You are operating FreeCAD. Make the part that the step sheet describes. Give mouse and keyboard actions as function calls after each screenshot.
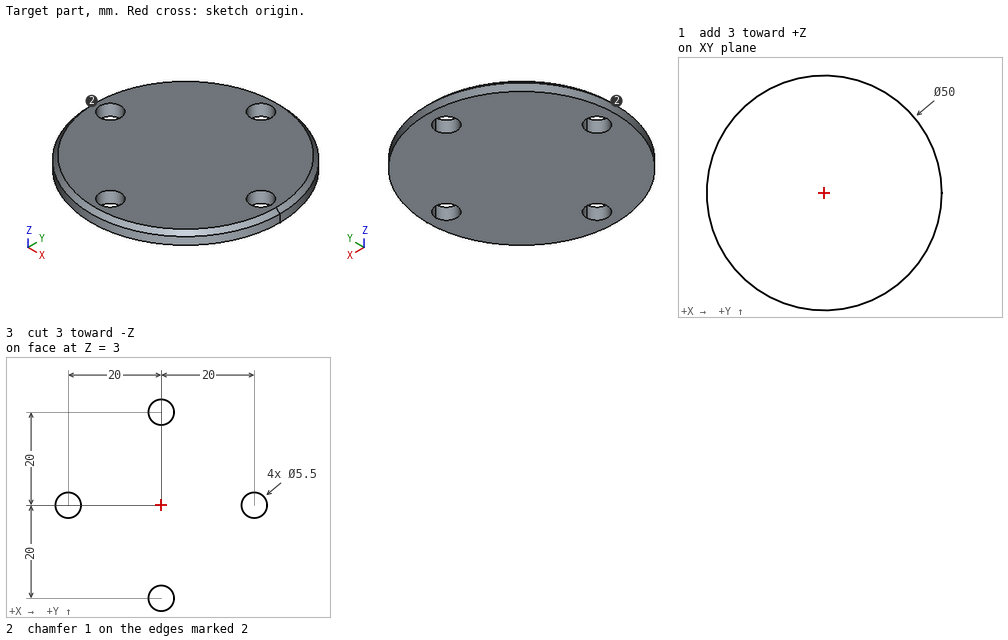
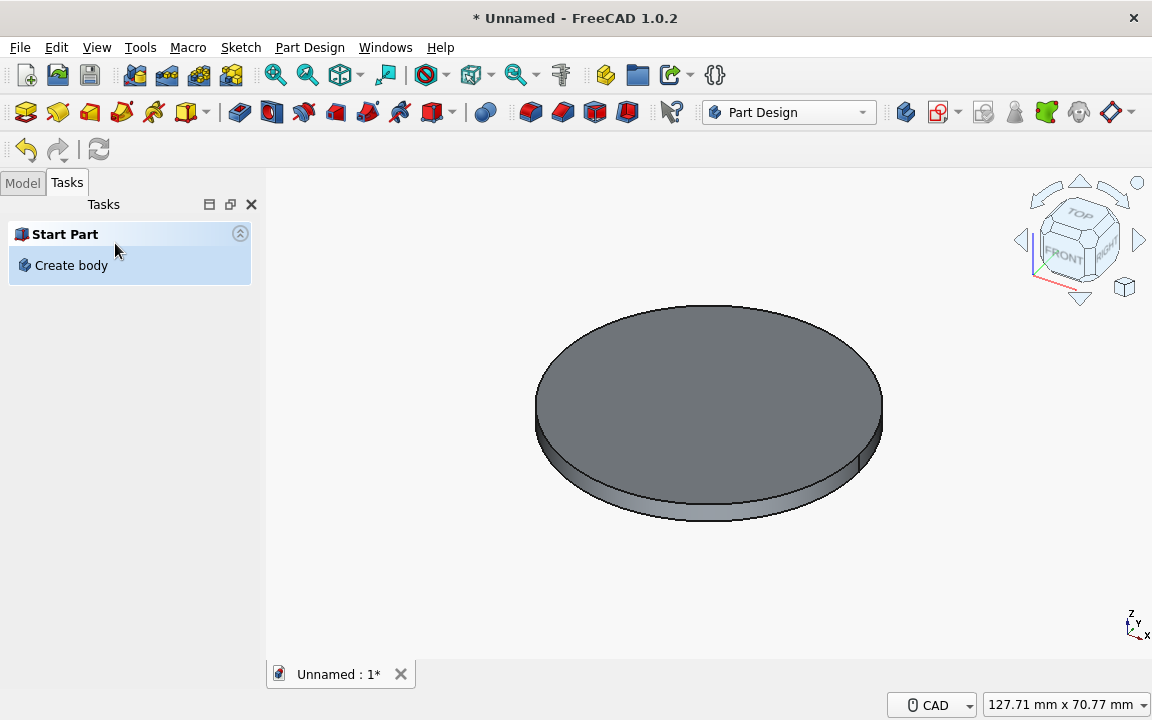
click(537, 414)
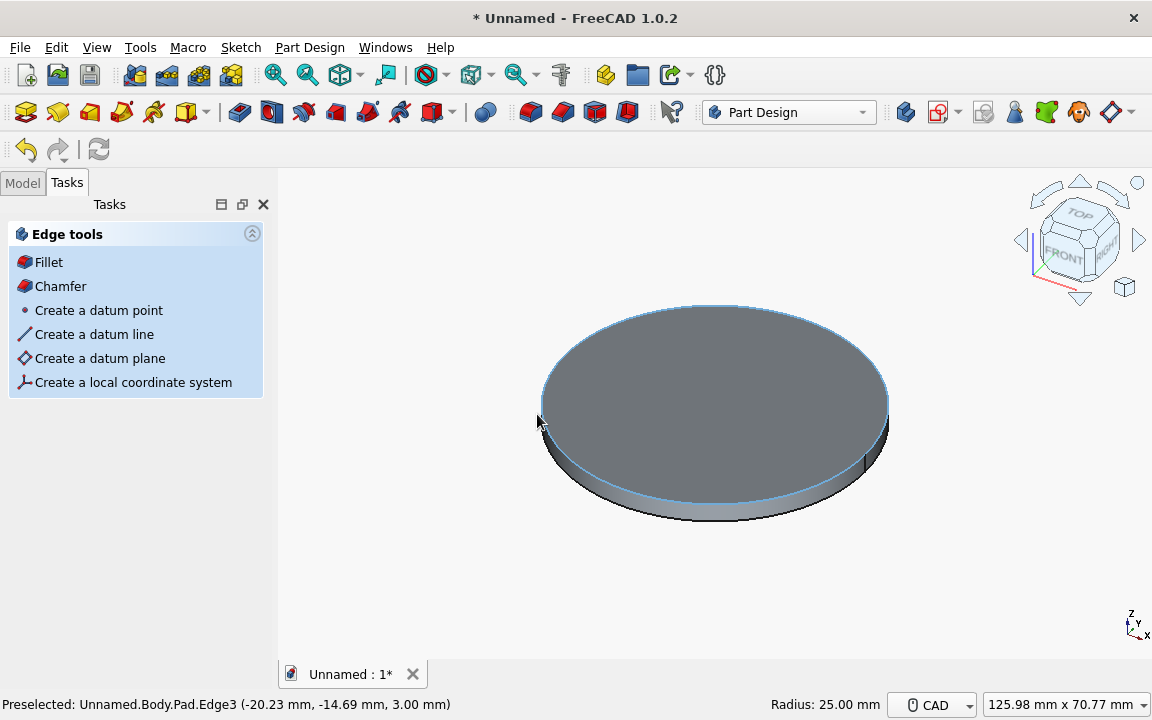
click(564, 112)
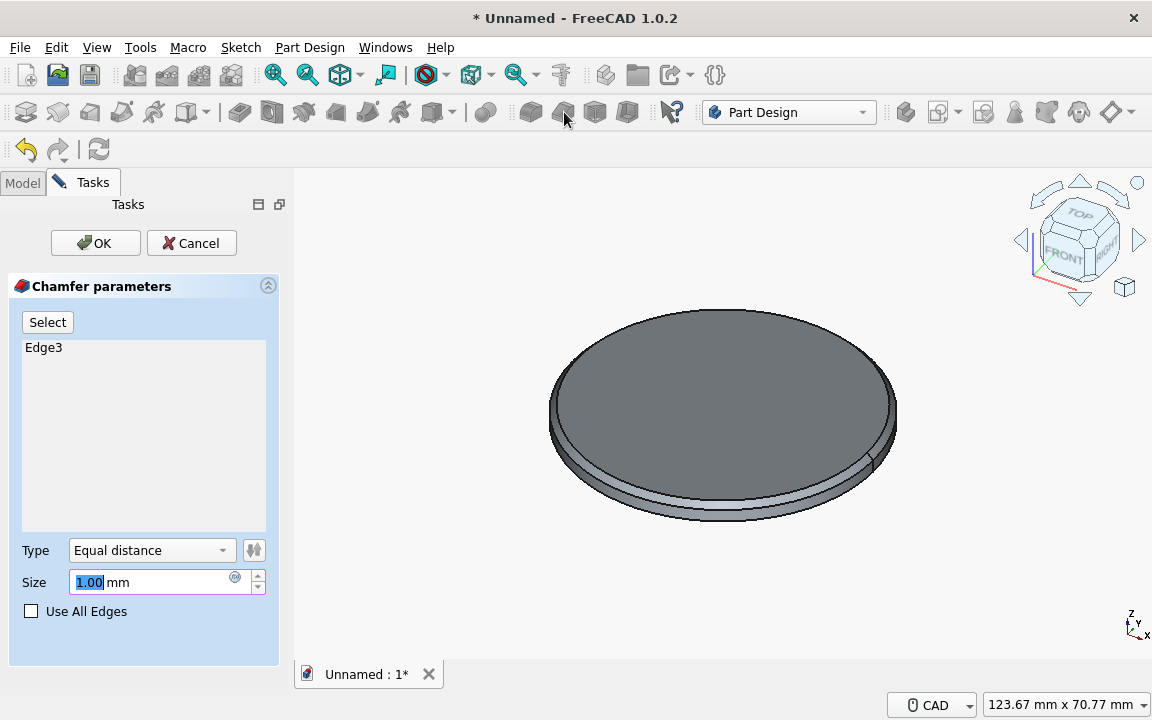
text(1)
key(Tab)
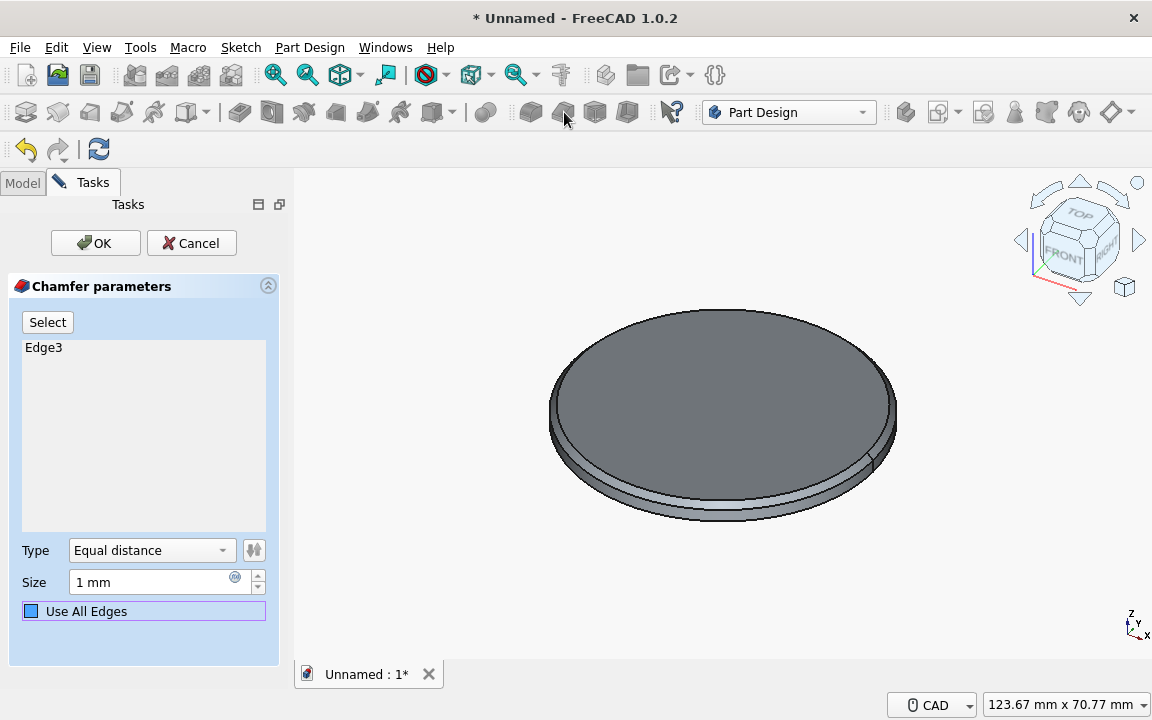
click(96, 243)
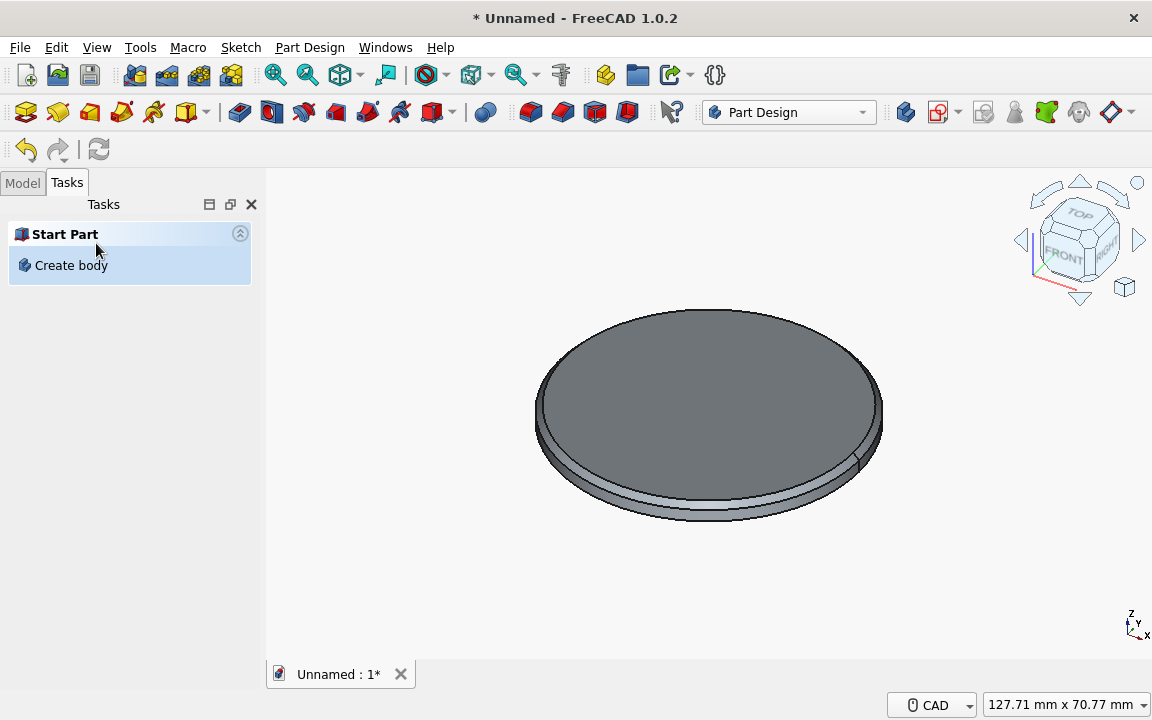
click(709, 404)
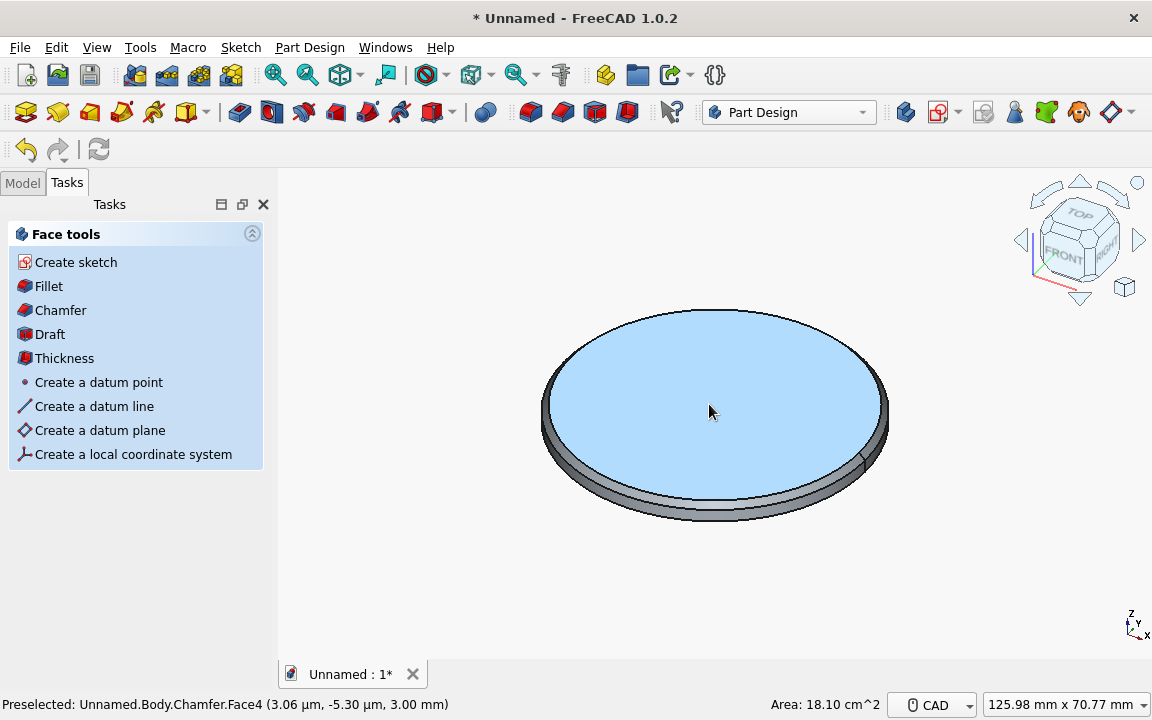
click(938, 112)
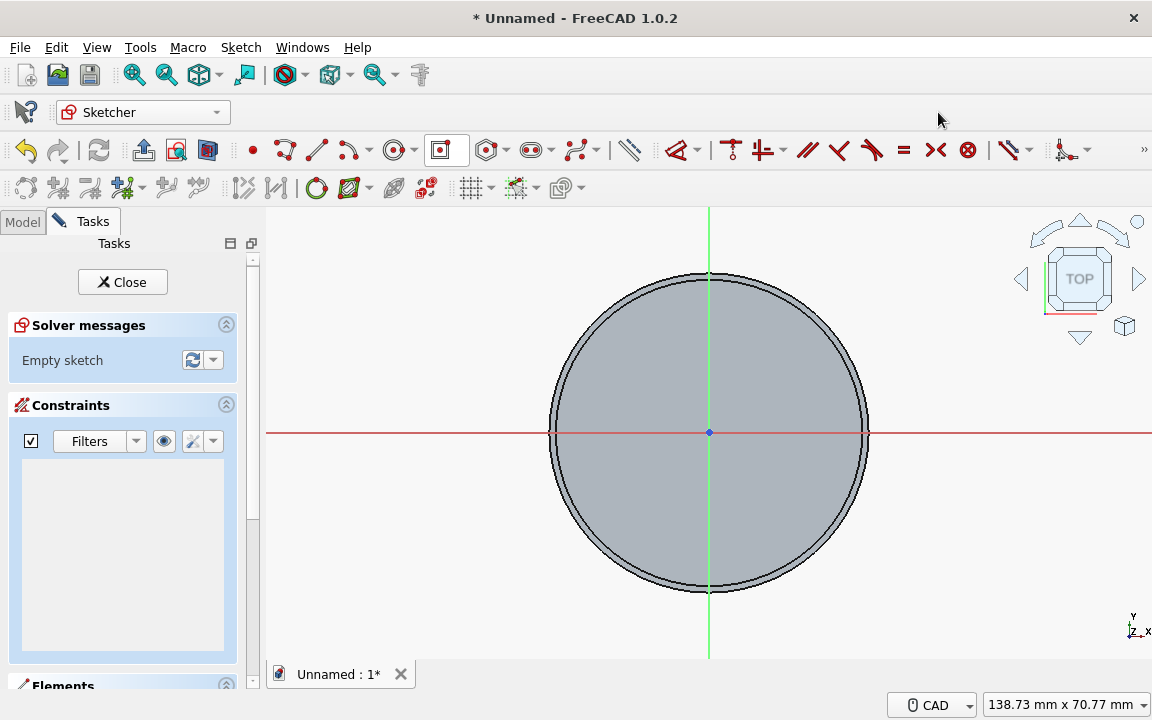
click(394, 150)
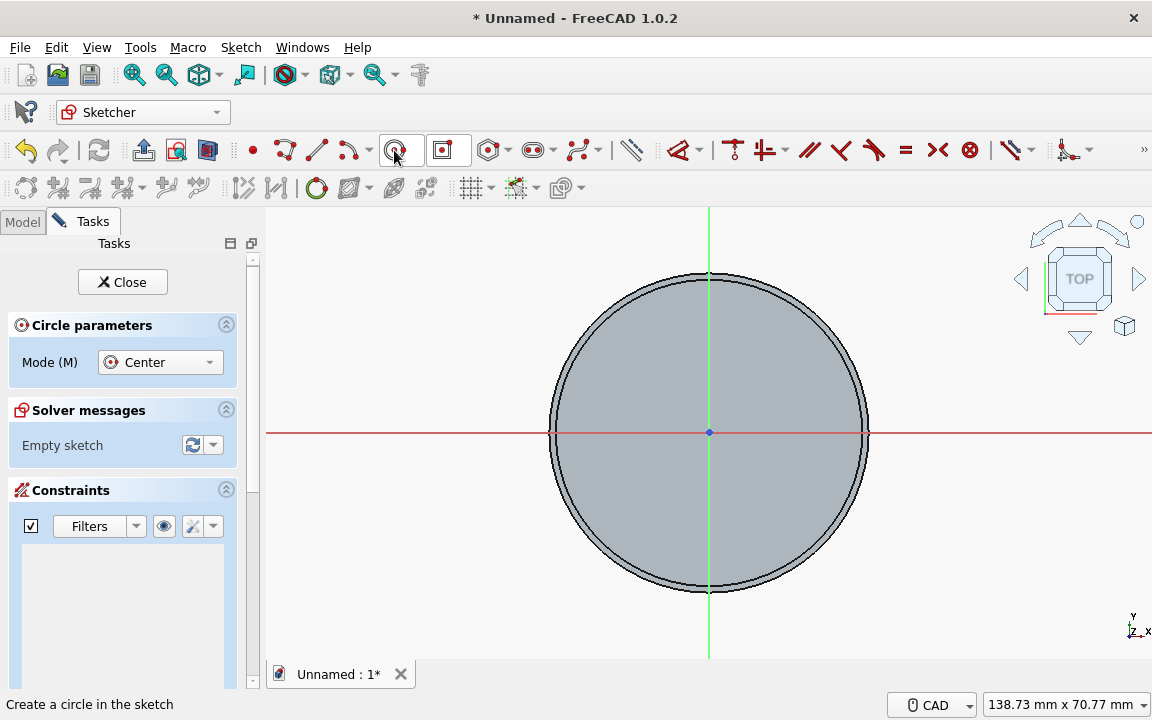
scroll(837, 433, up, 2)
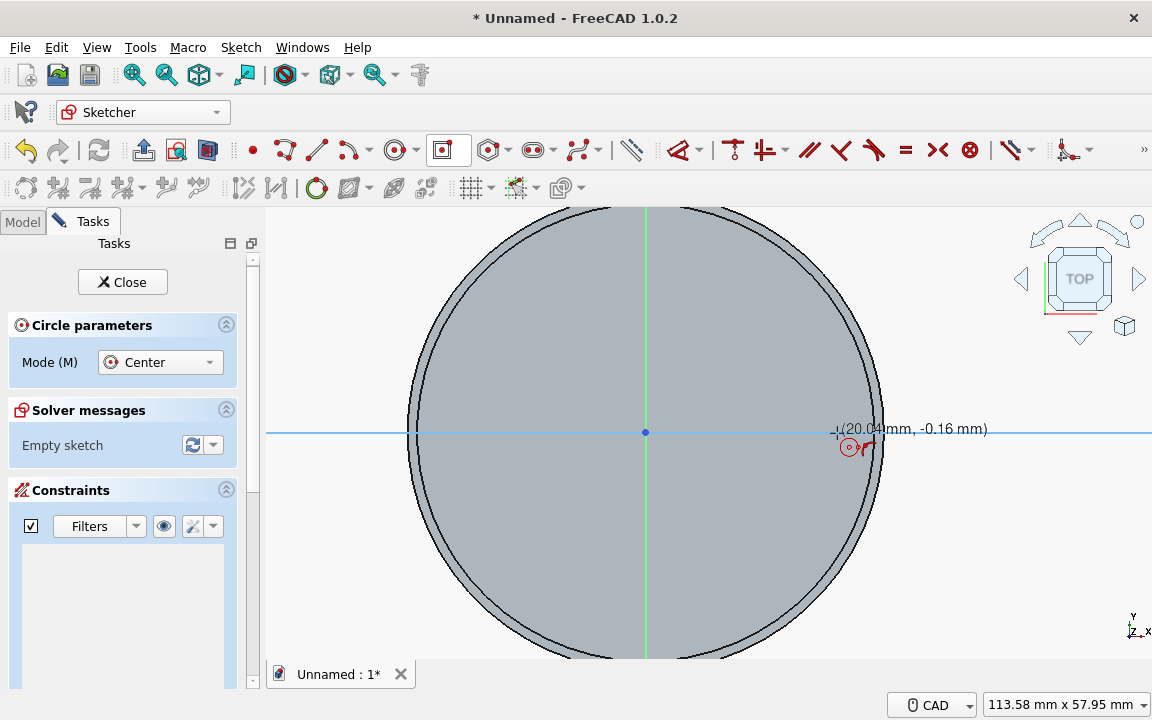
click(836, 433)
move(855, 414)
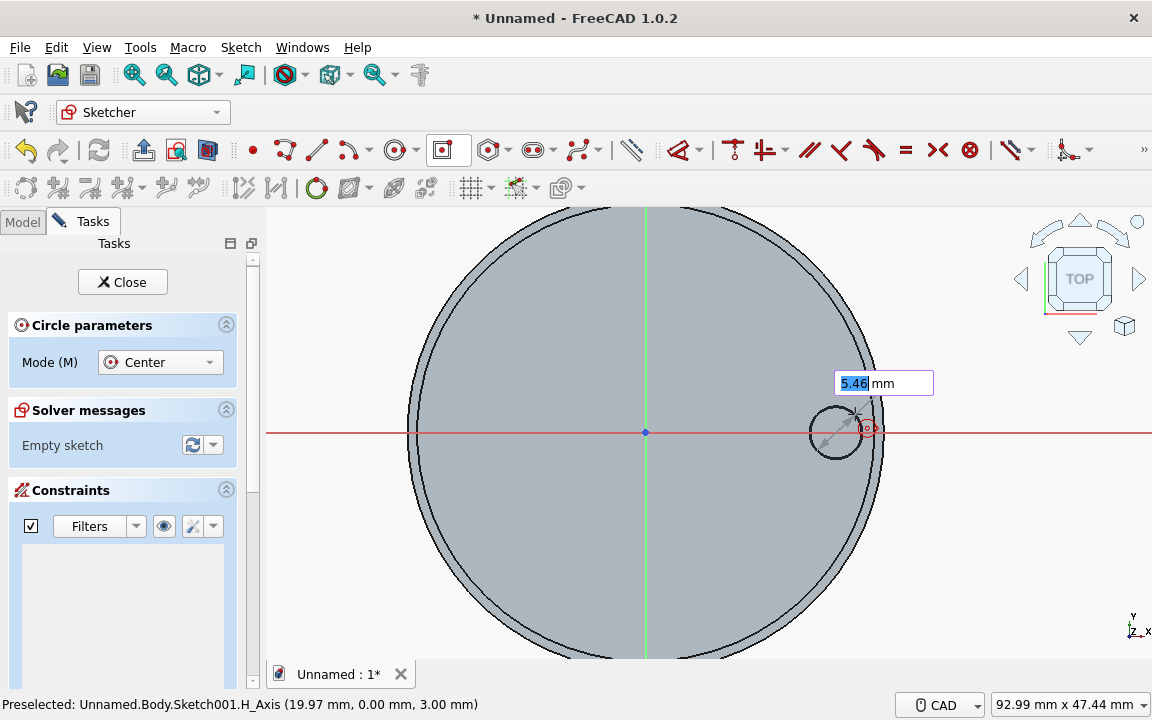
text(5.5)
key(Return)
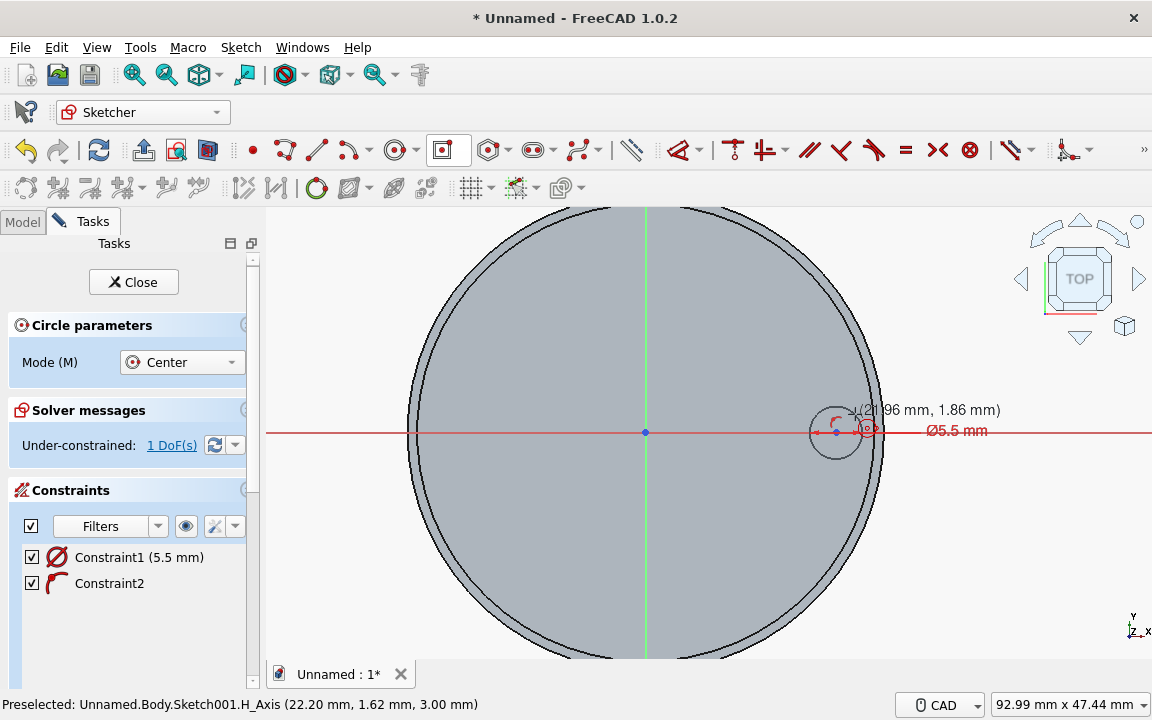
click(646, 623)
move(664, 605)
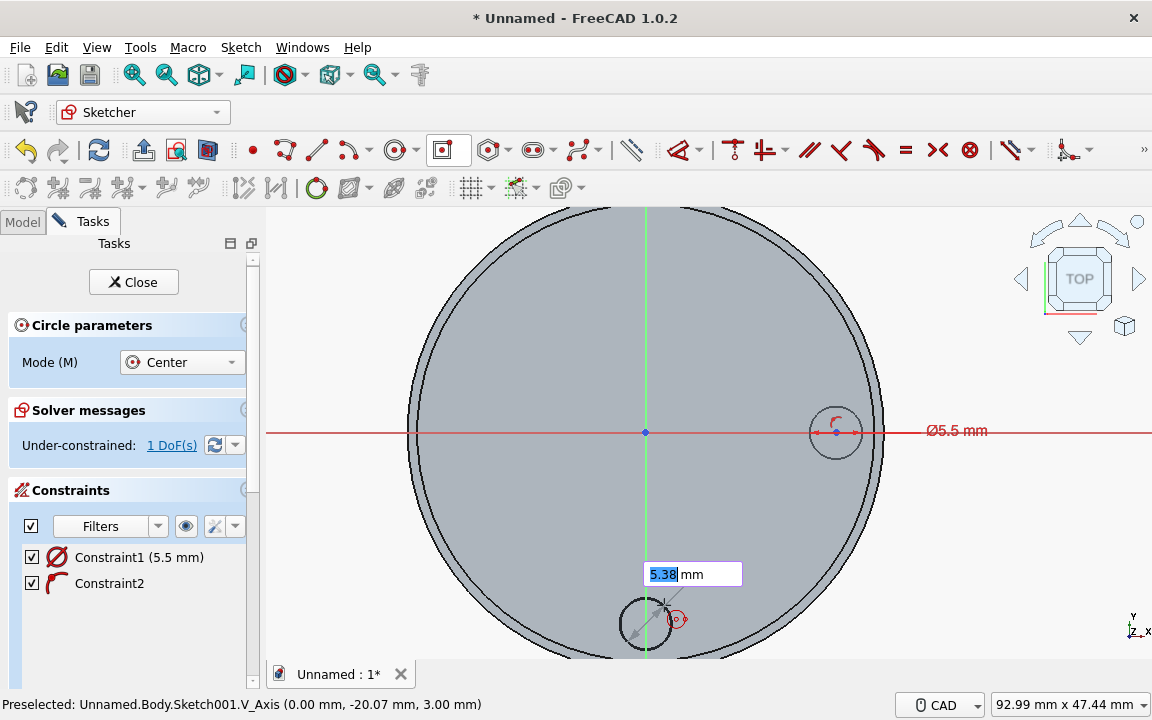
text(5.5)
key(Return)